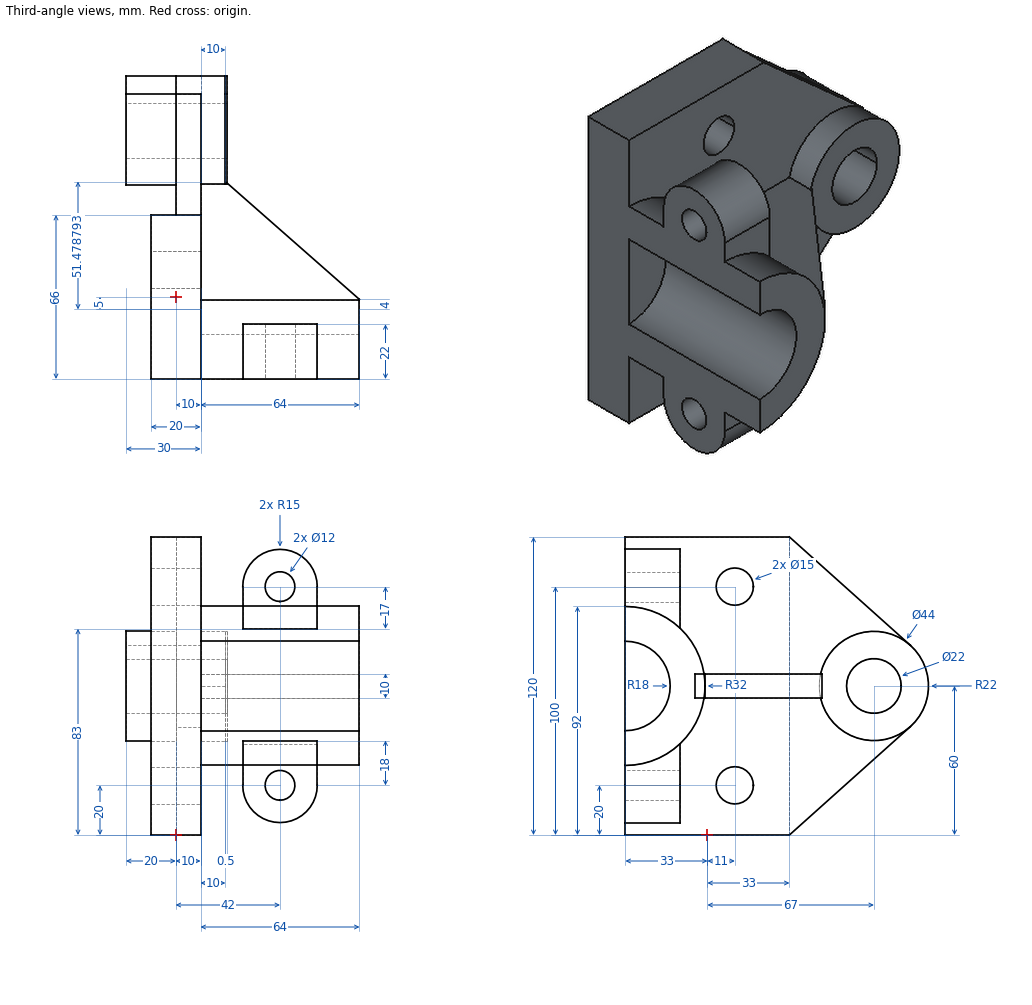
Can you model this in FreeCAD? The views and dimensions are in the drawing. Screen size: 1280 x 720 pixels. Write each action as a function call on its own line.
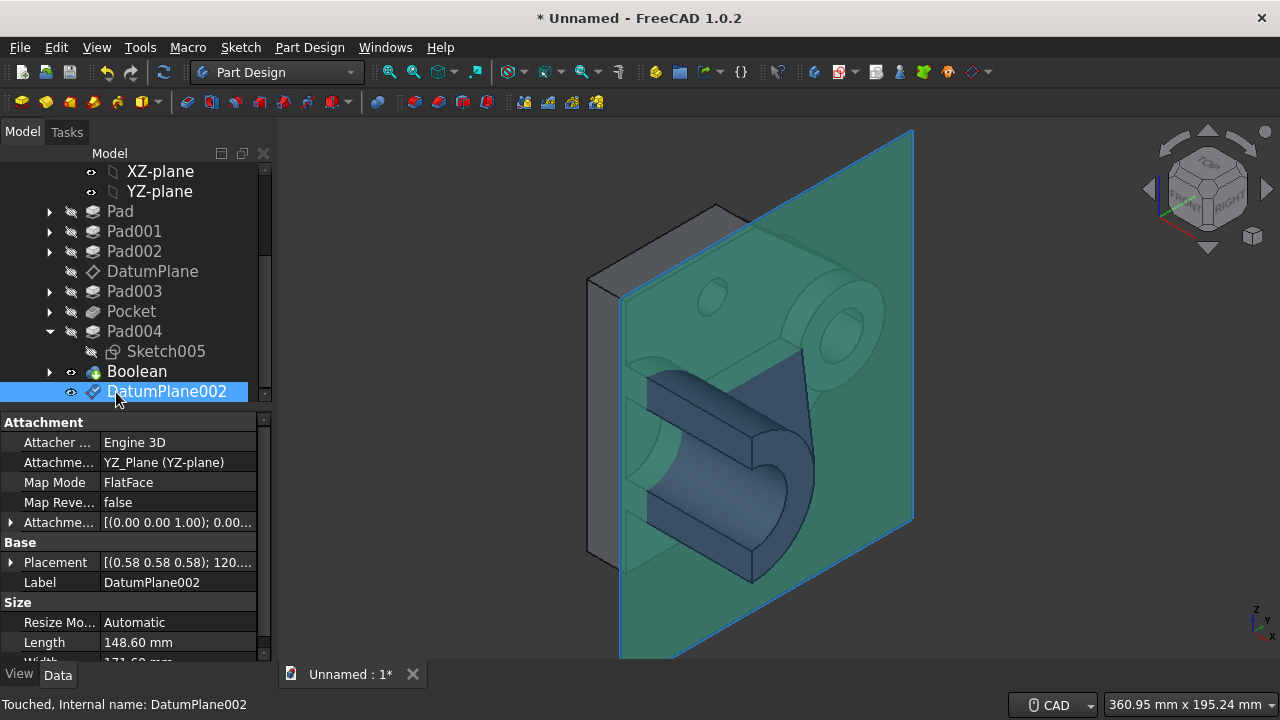
click(840, 72)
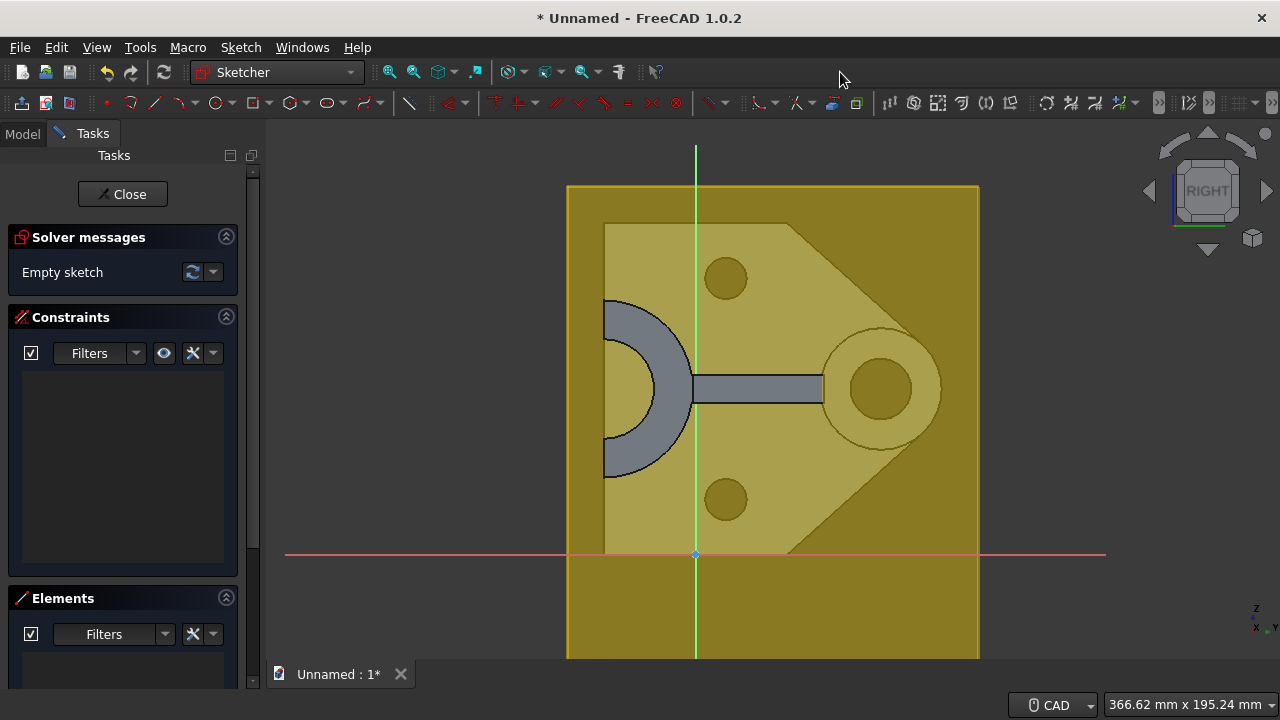
click(70, 104)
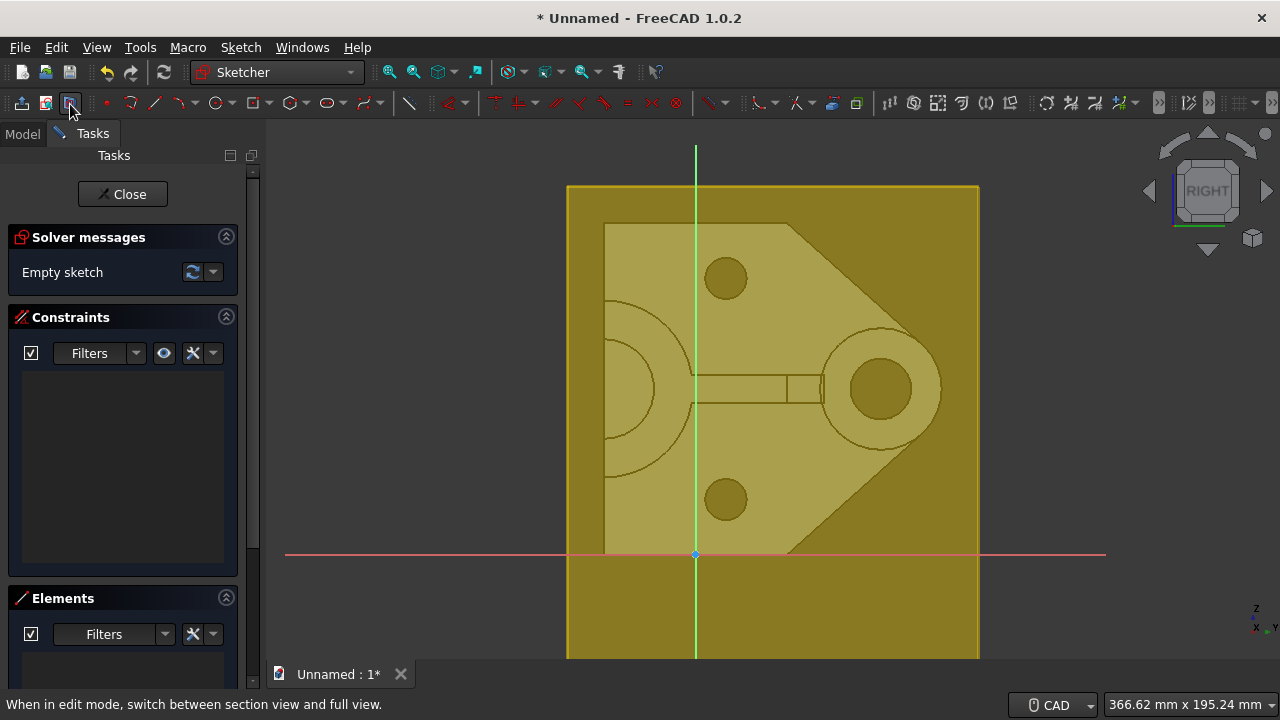
scroll(1051, 548, up, 2)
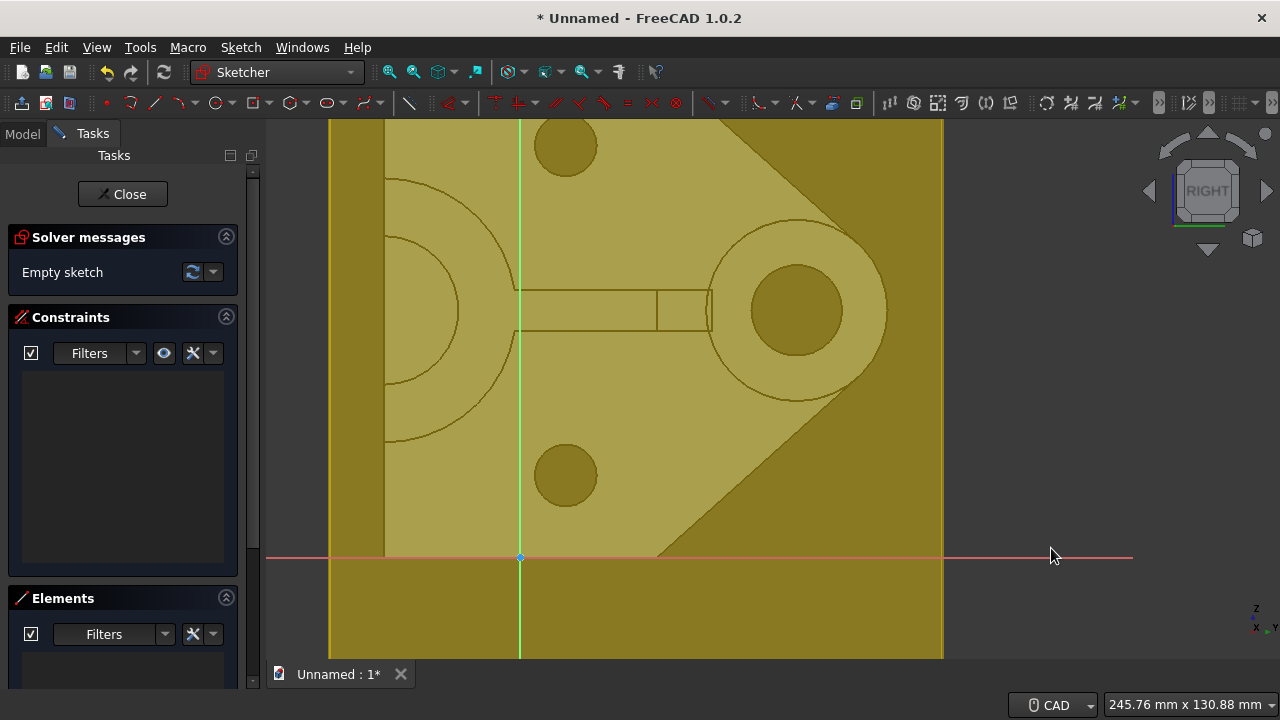
click(216, 104)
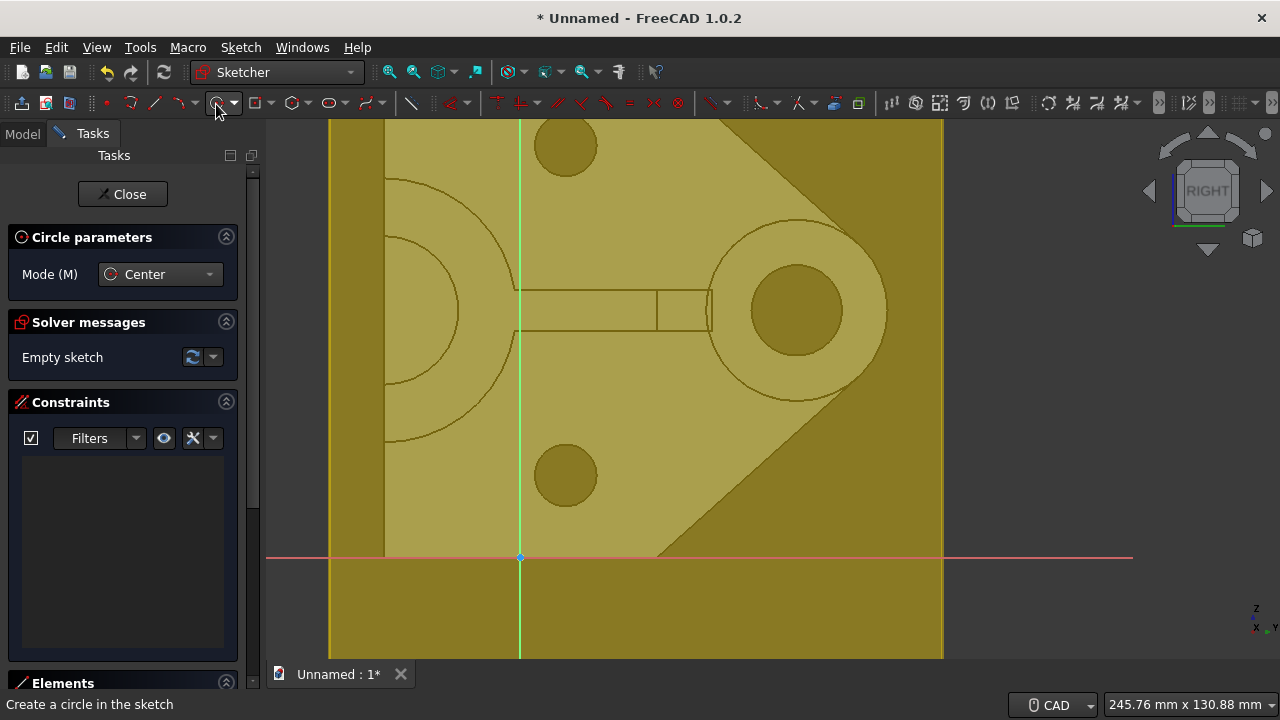
click(797, 310)
click(861, 246)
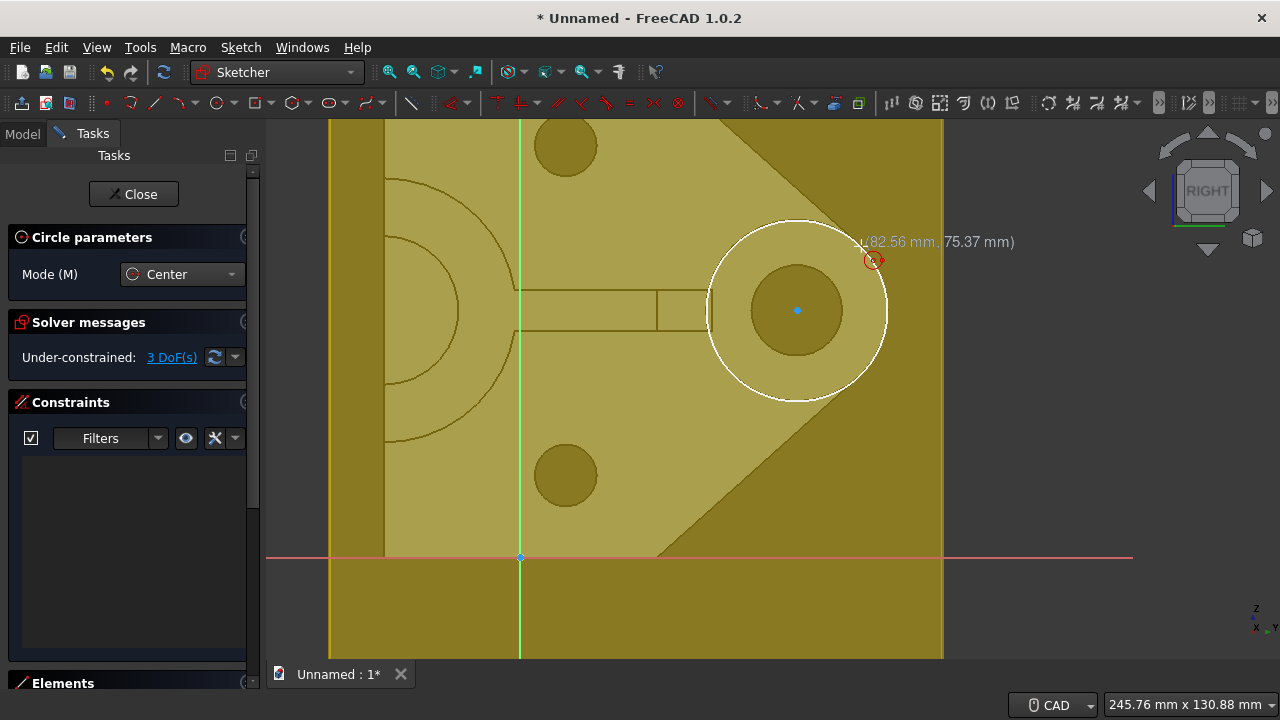
click(797, 311)
click(829, 278)
key(Escape)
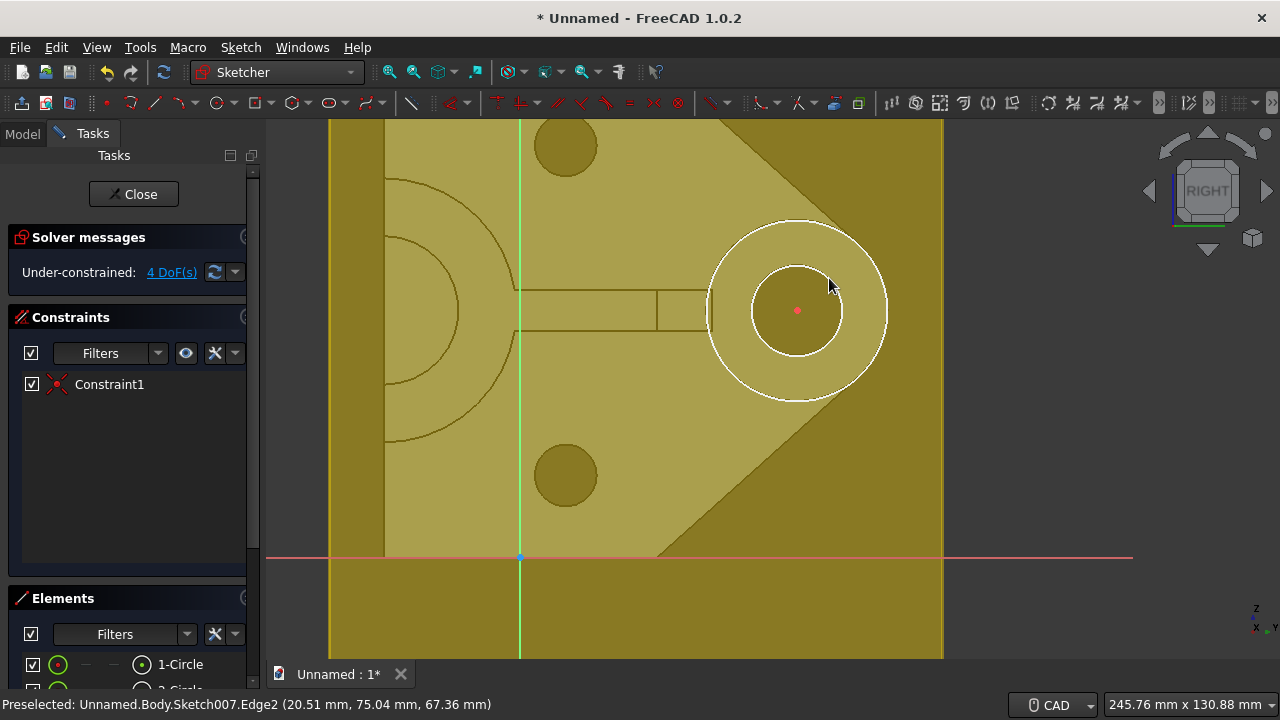
click(450, 104)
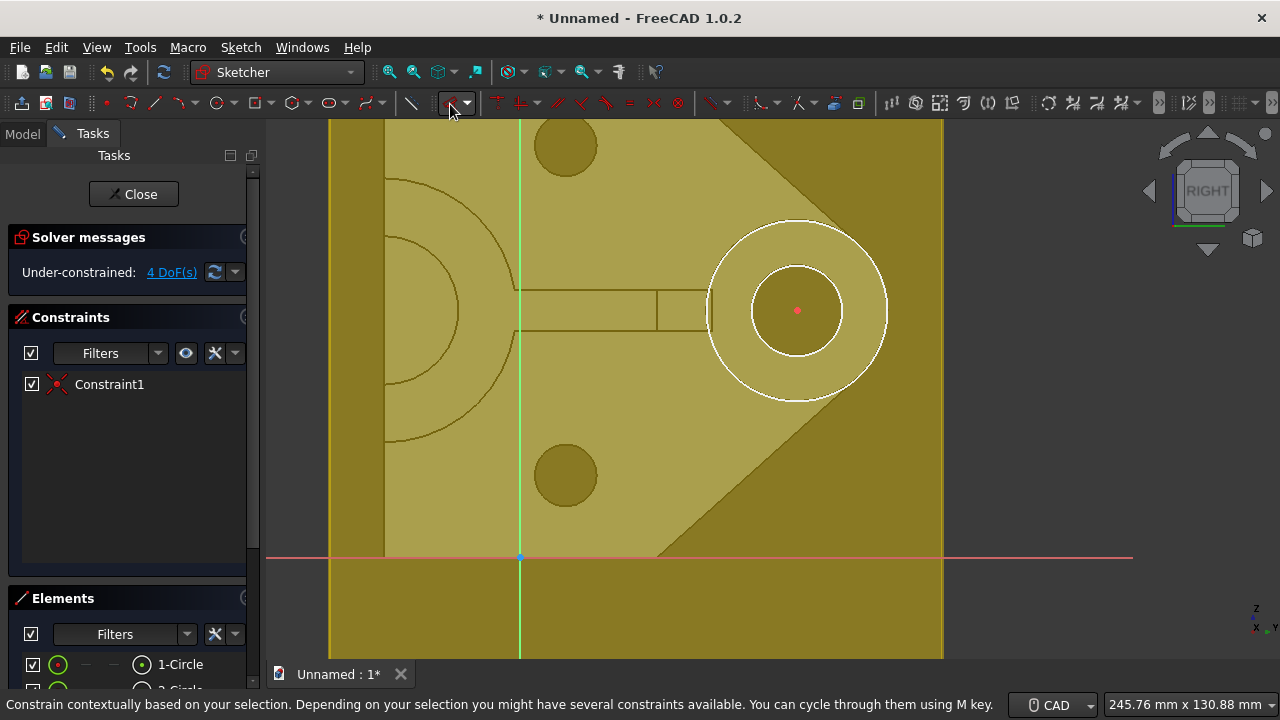
click(861, 247)
click(884, 224)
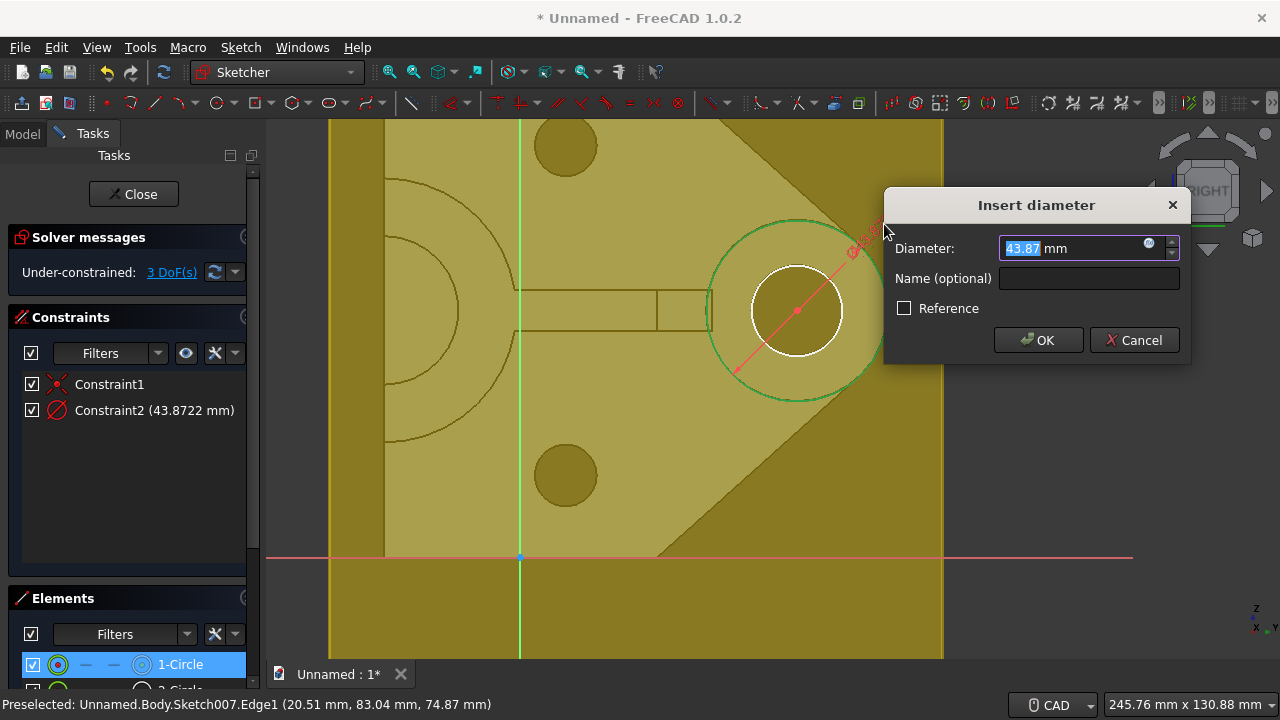
text(44)
key(Return)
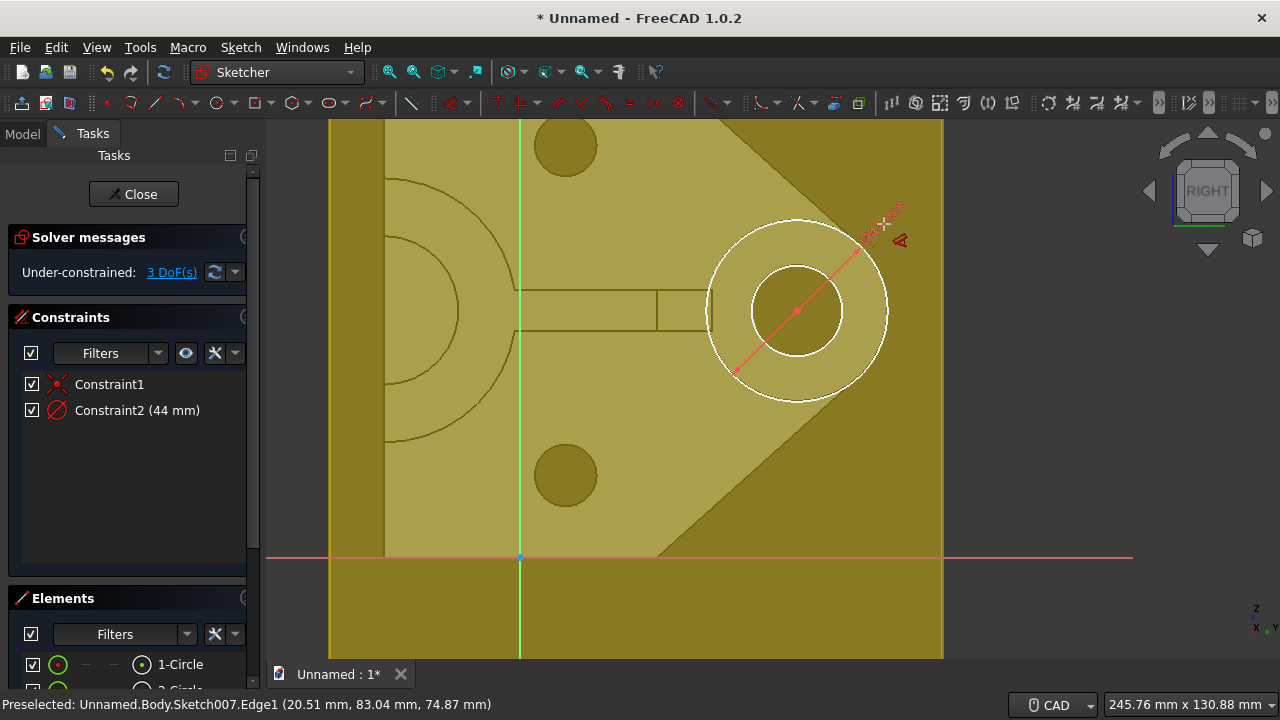
click(829, 279)
click(852, 256)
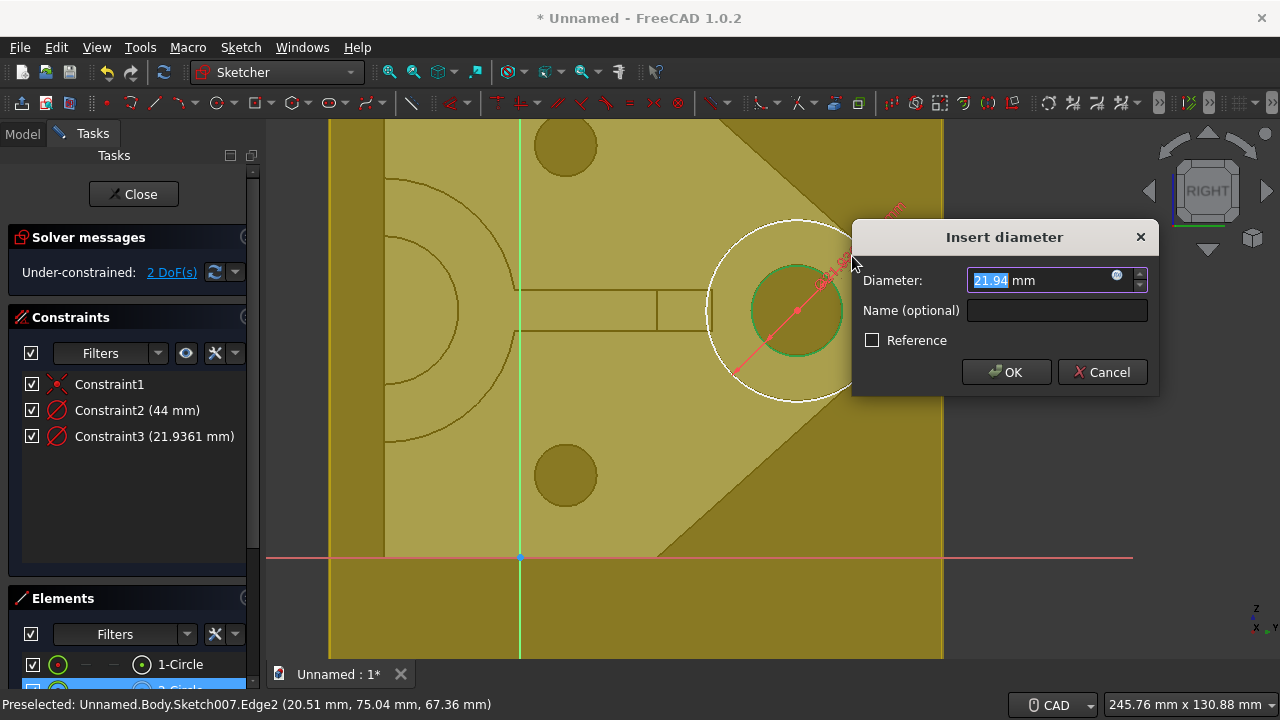
text(22)
key(Return)